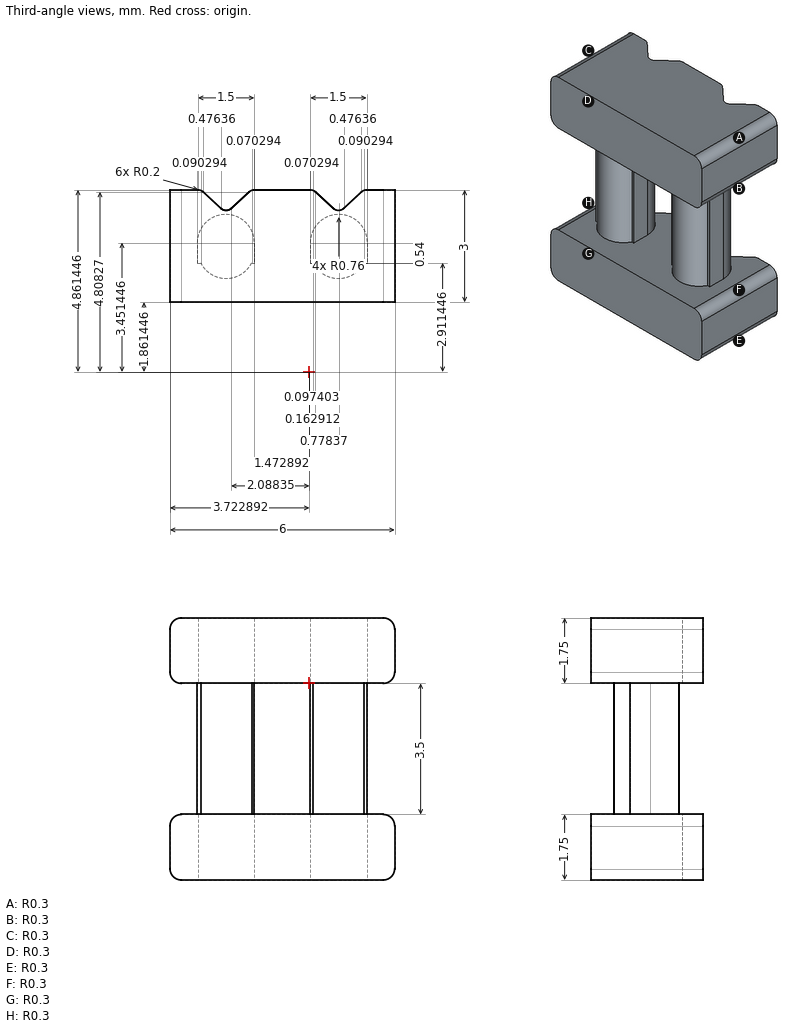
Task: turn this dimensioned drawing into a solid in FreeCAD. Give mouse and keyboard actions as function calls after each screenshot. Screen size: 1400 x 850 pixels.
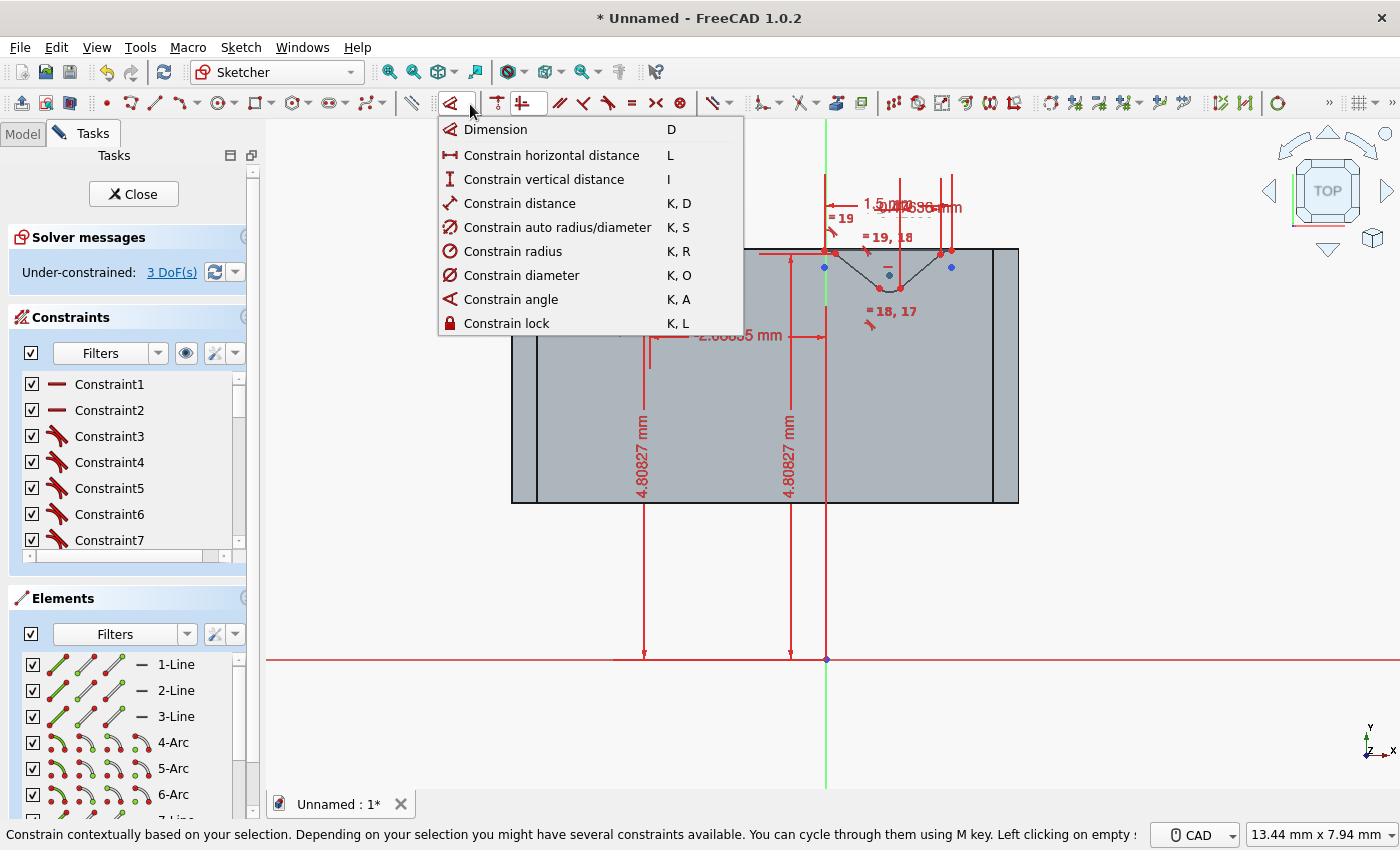
click(591, 155)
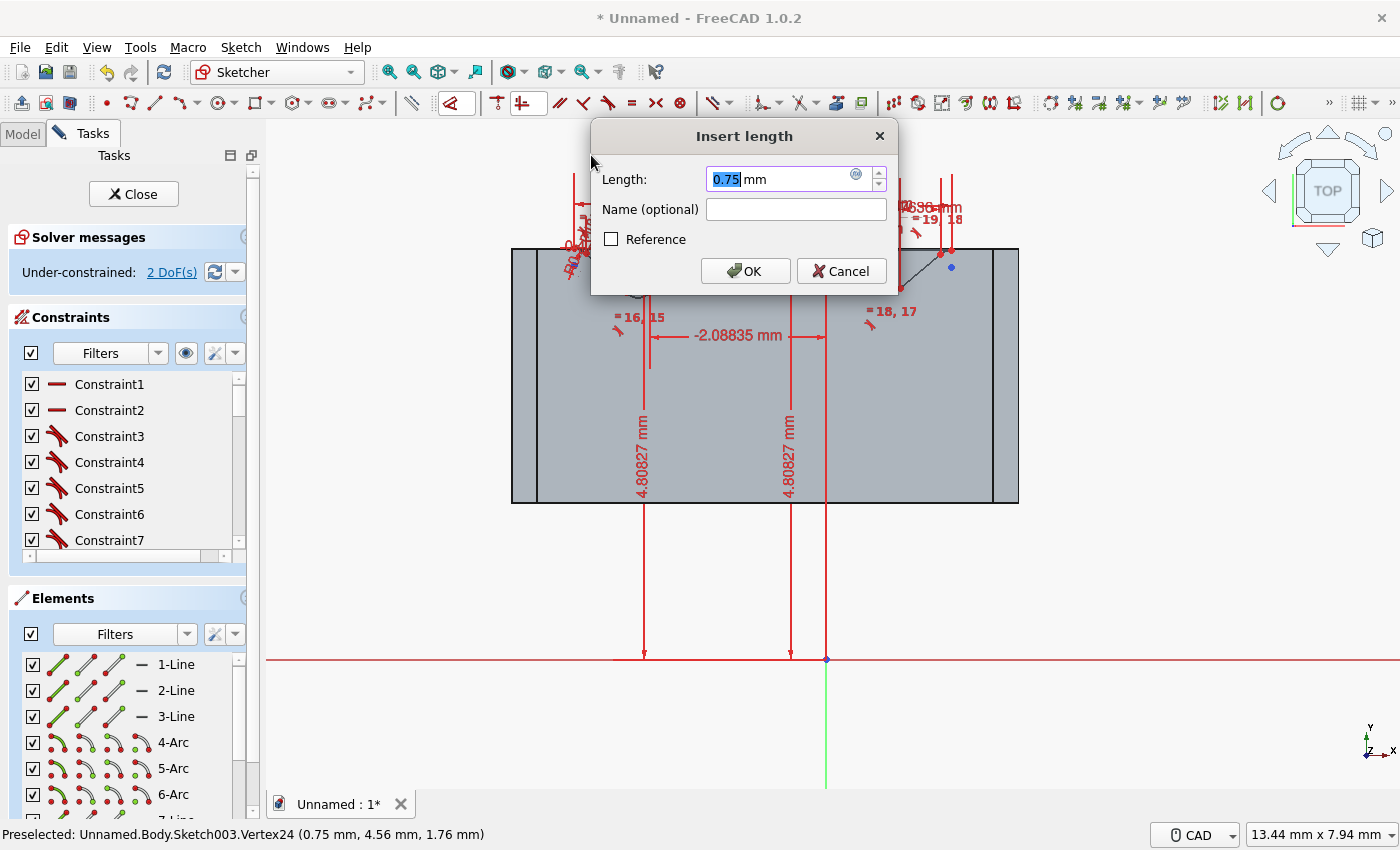
text(0.77837)
key(Return)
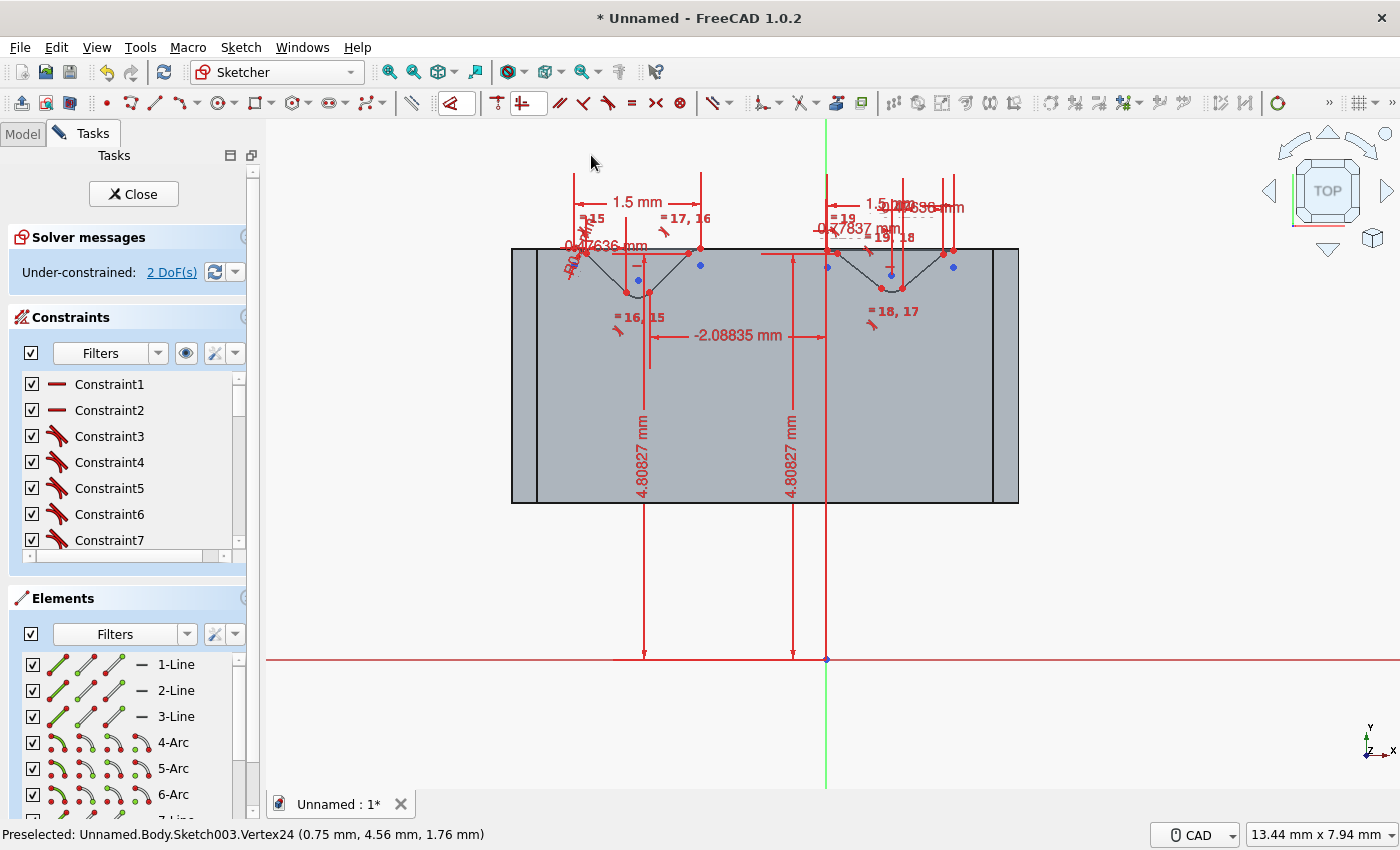
click(701, 249)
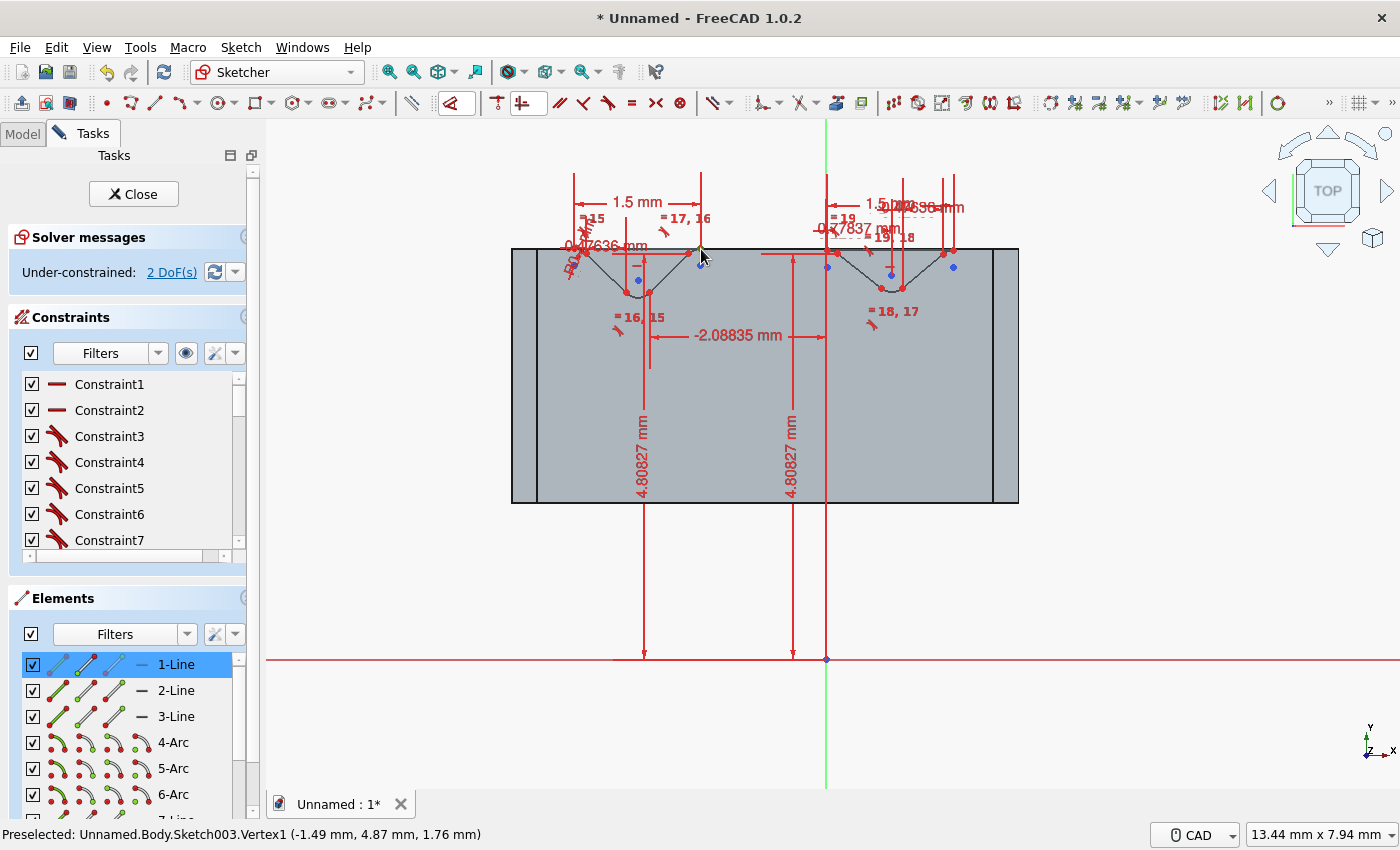
click(470, 104)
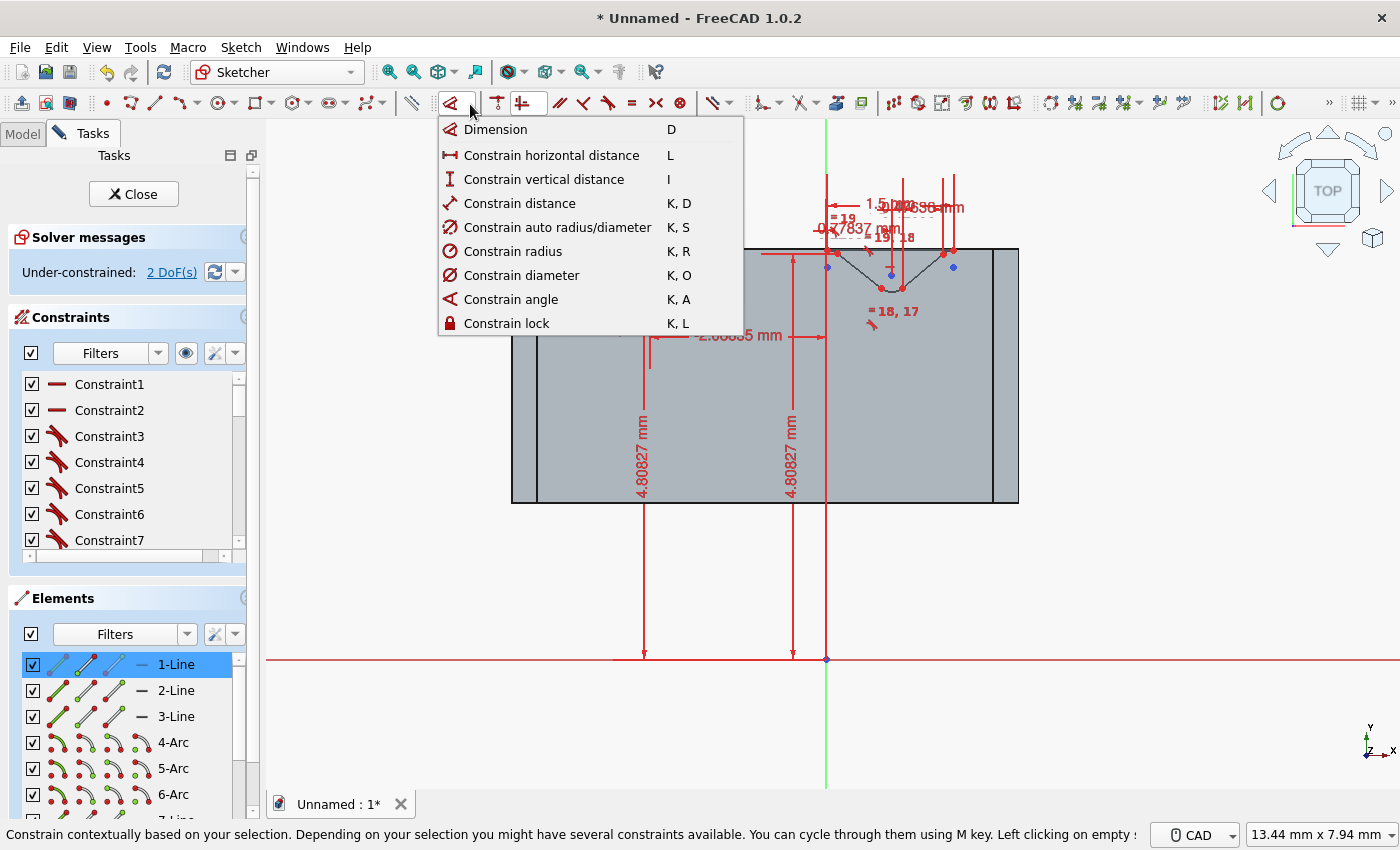
click(591, 155)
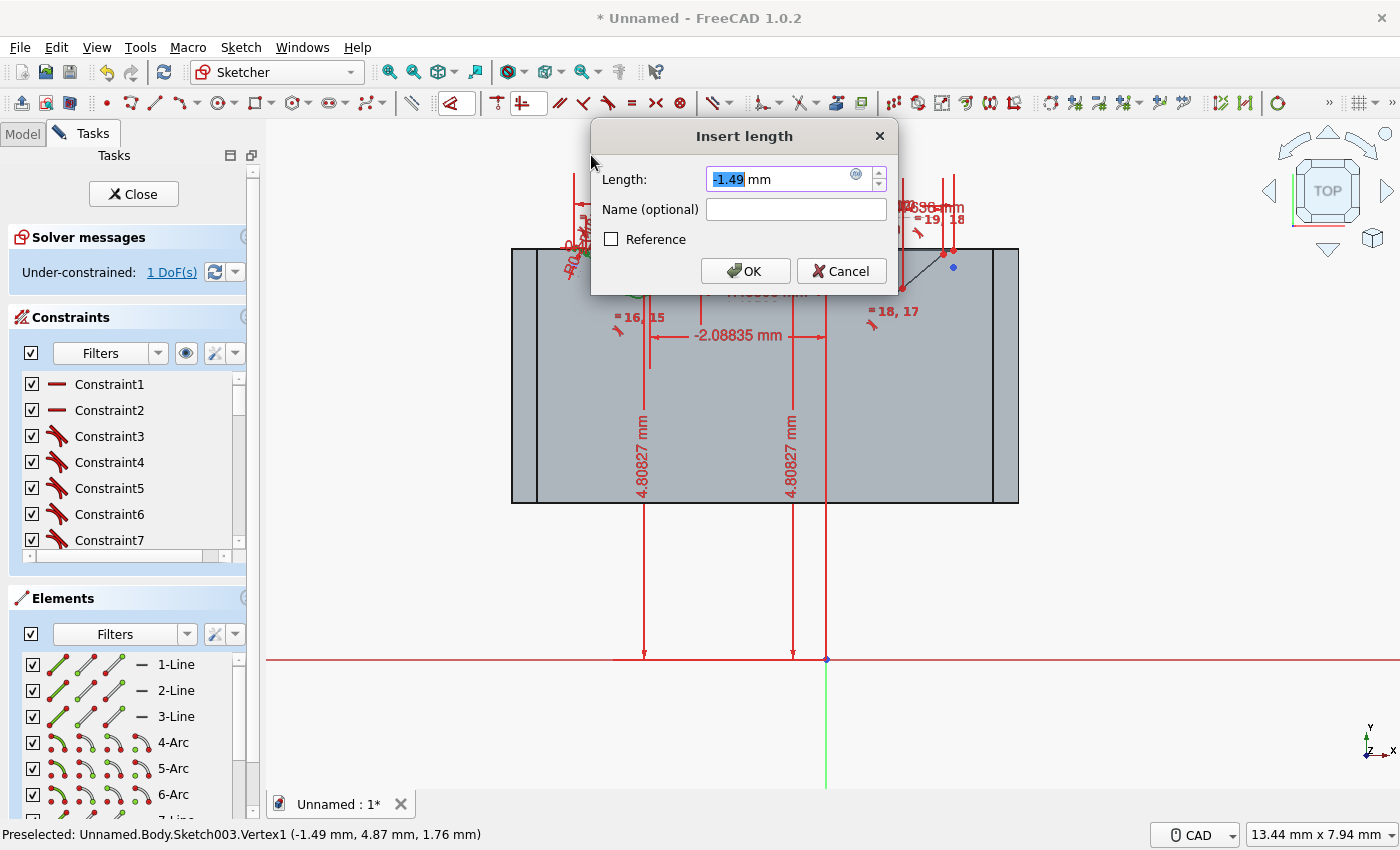
text(-1.472892)
key(Return)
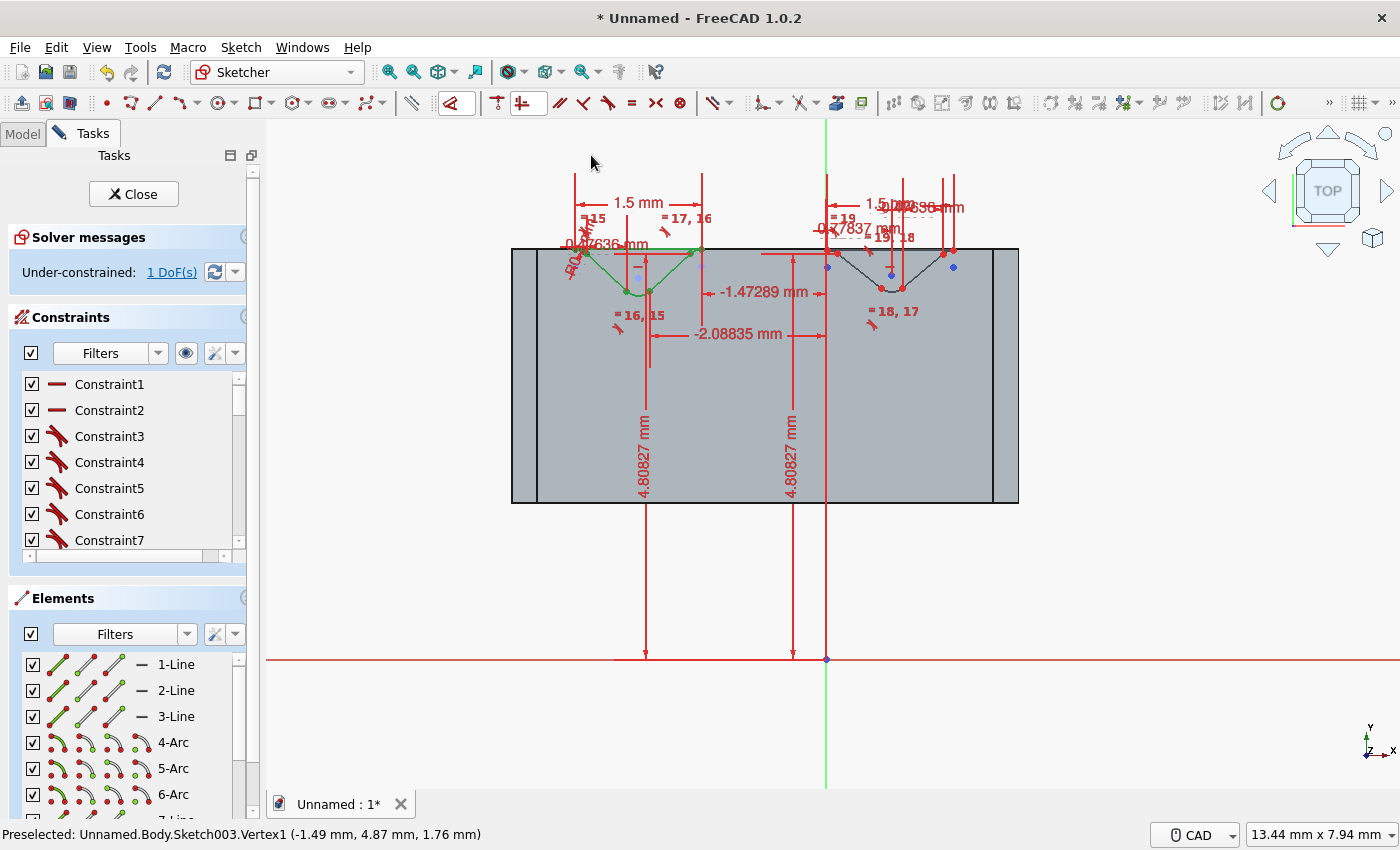
scroll(838, 254, up, 6)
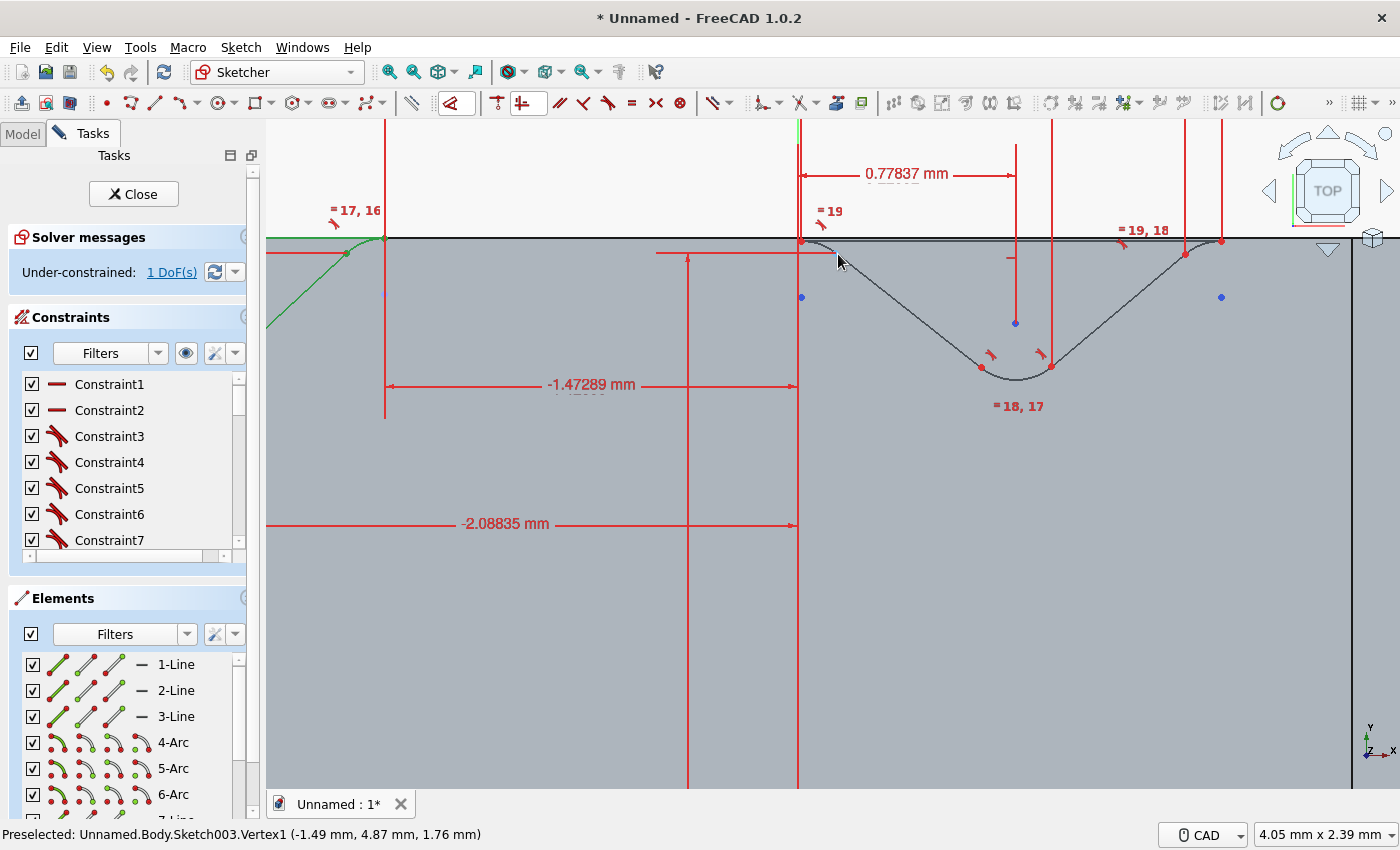
click(836, 253)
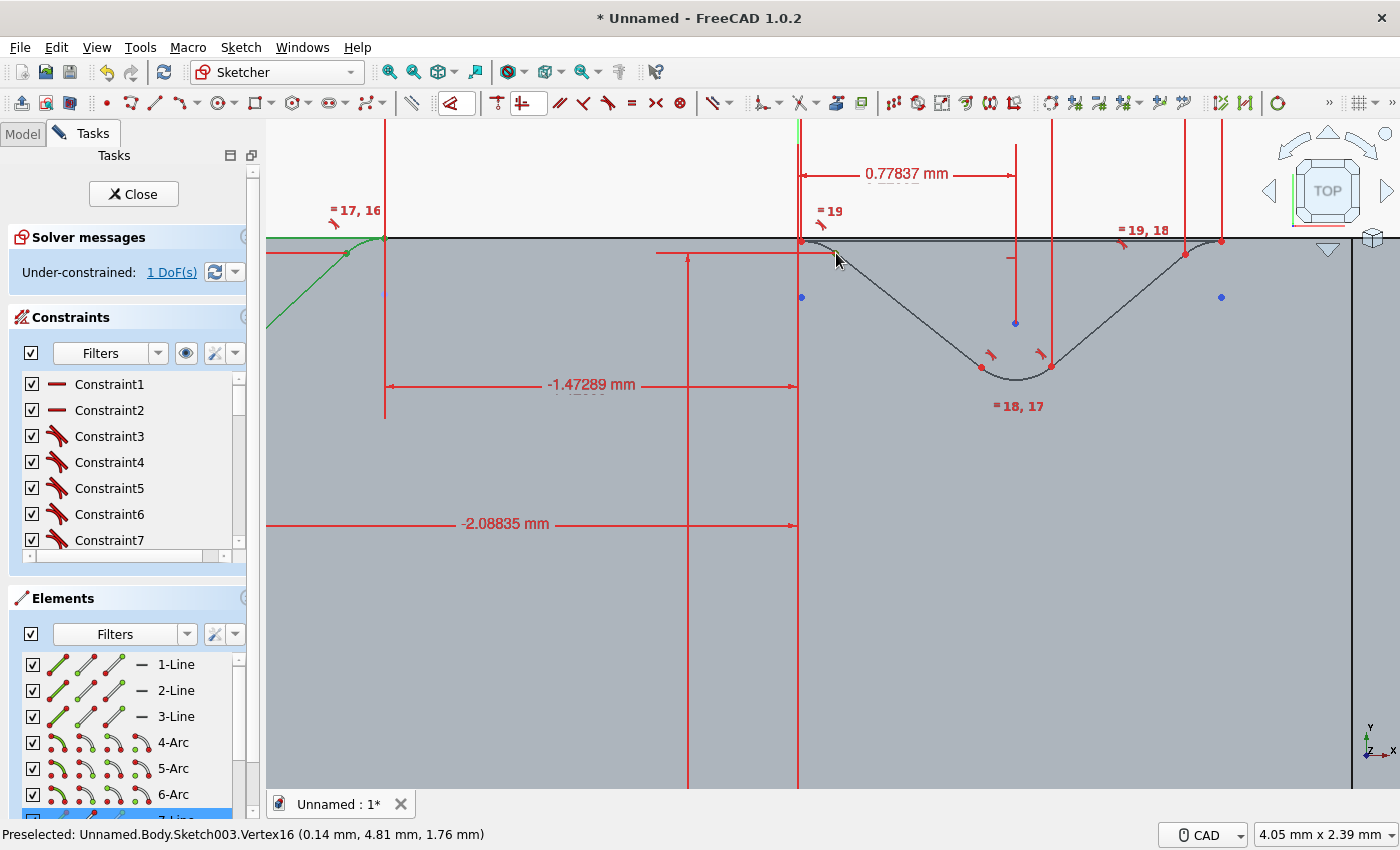
key(l)